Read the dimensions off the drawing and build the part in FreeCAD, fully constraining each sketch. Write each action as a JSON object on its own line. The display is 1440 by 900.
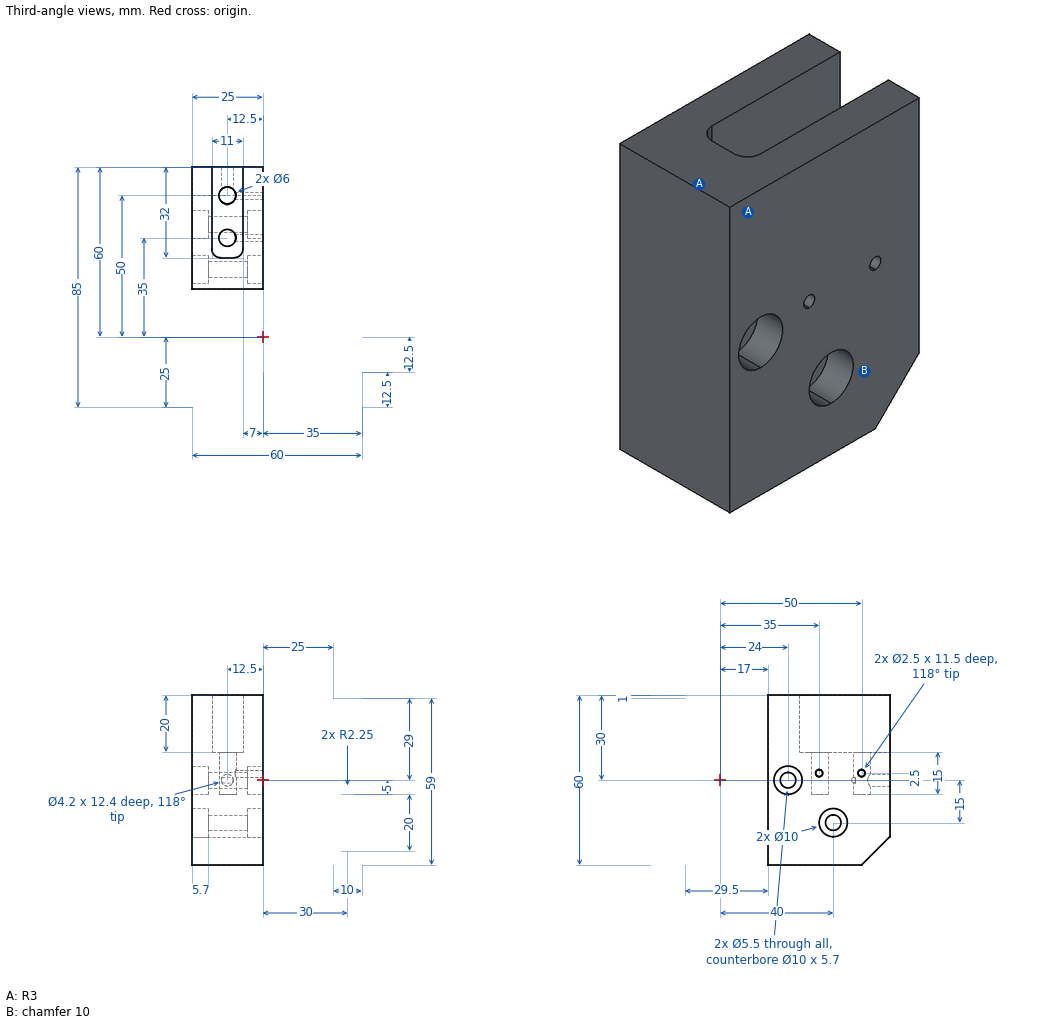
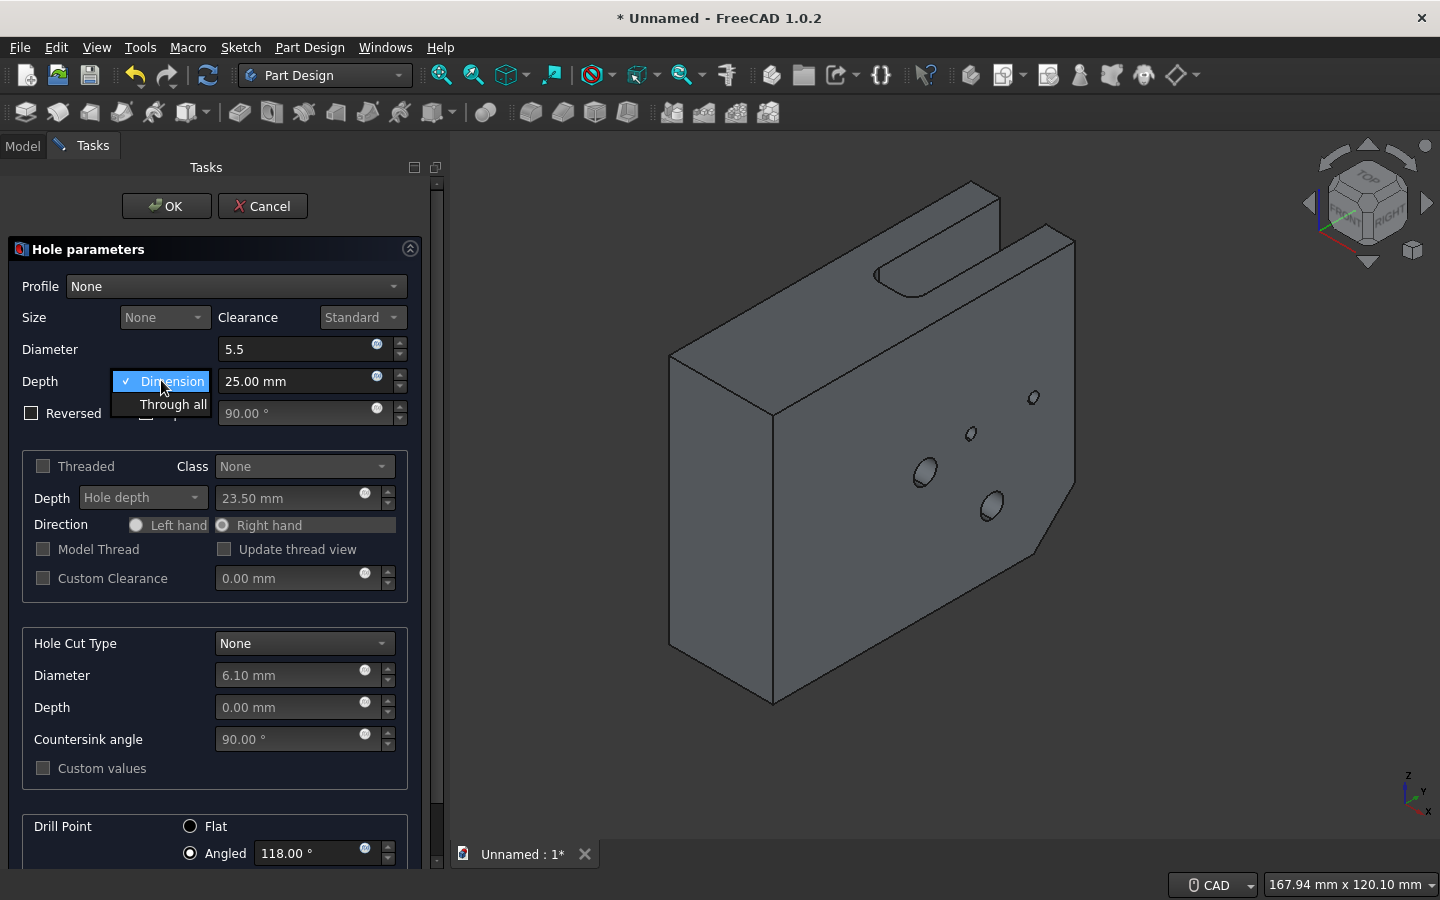
{"action": "left_click", "coordinate": [160, 404]}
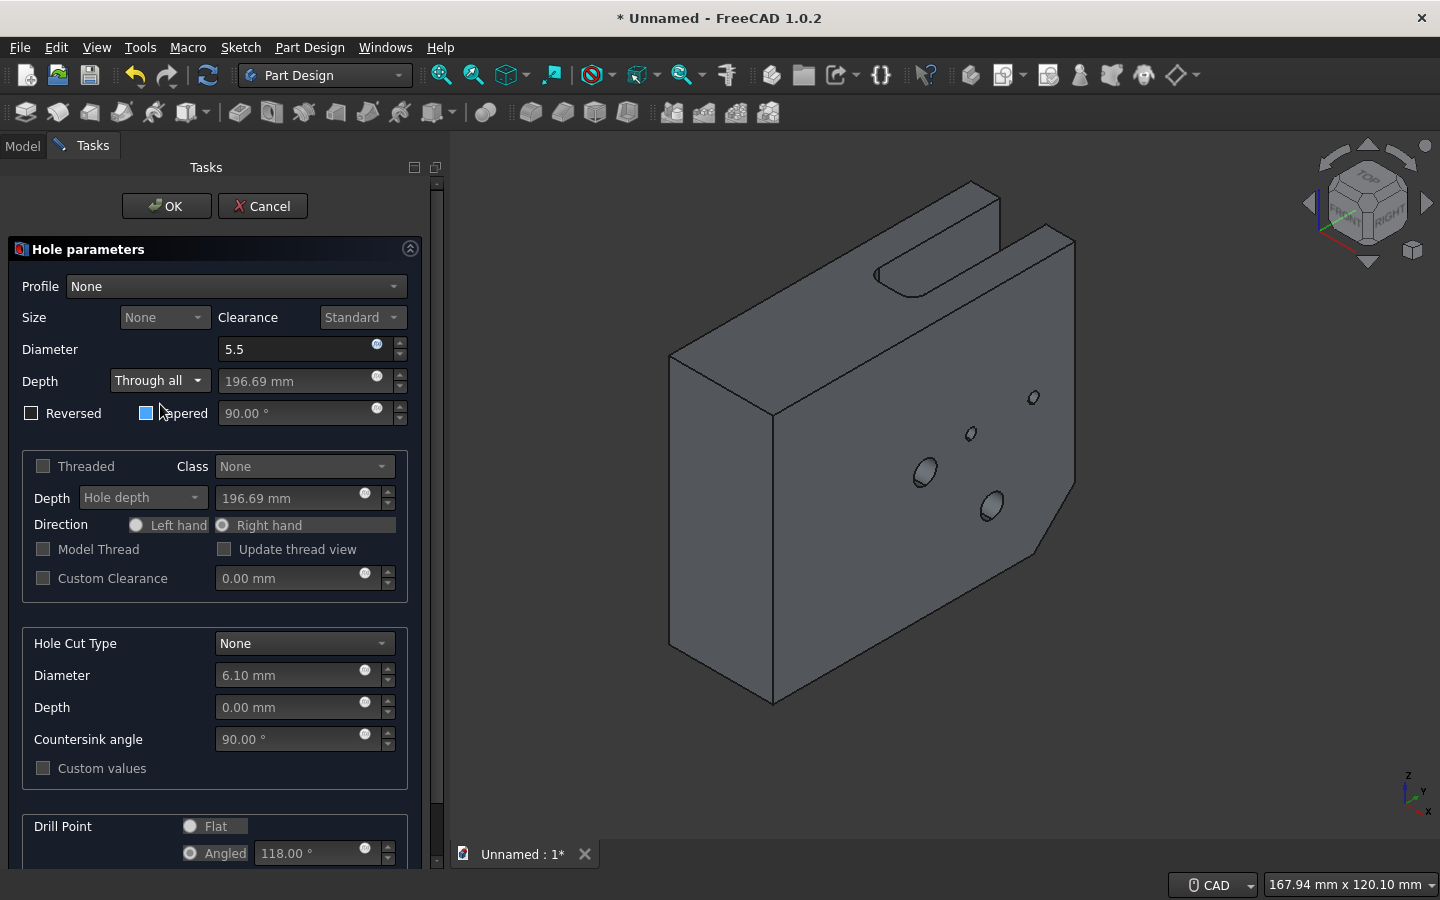
{"action": "left_click", "coordinate": [306, 644]}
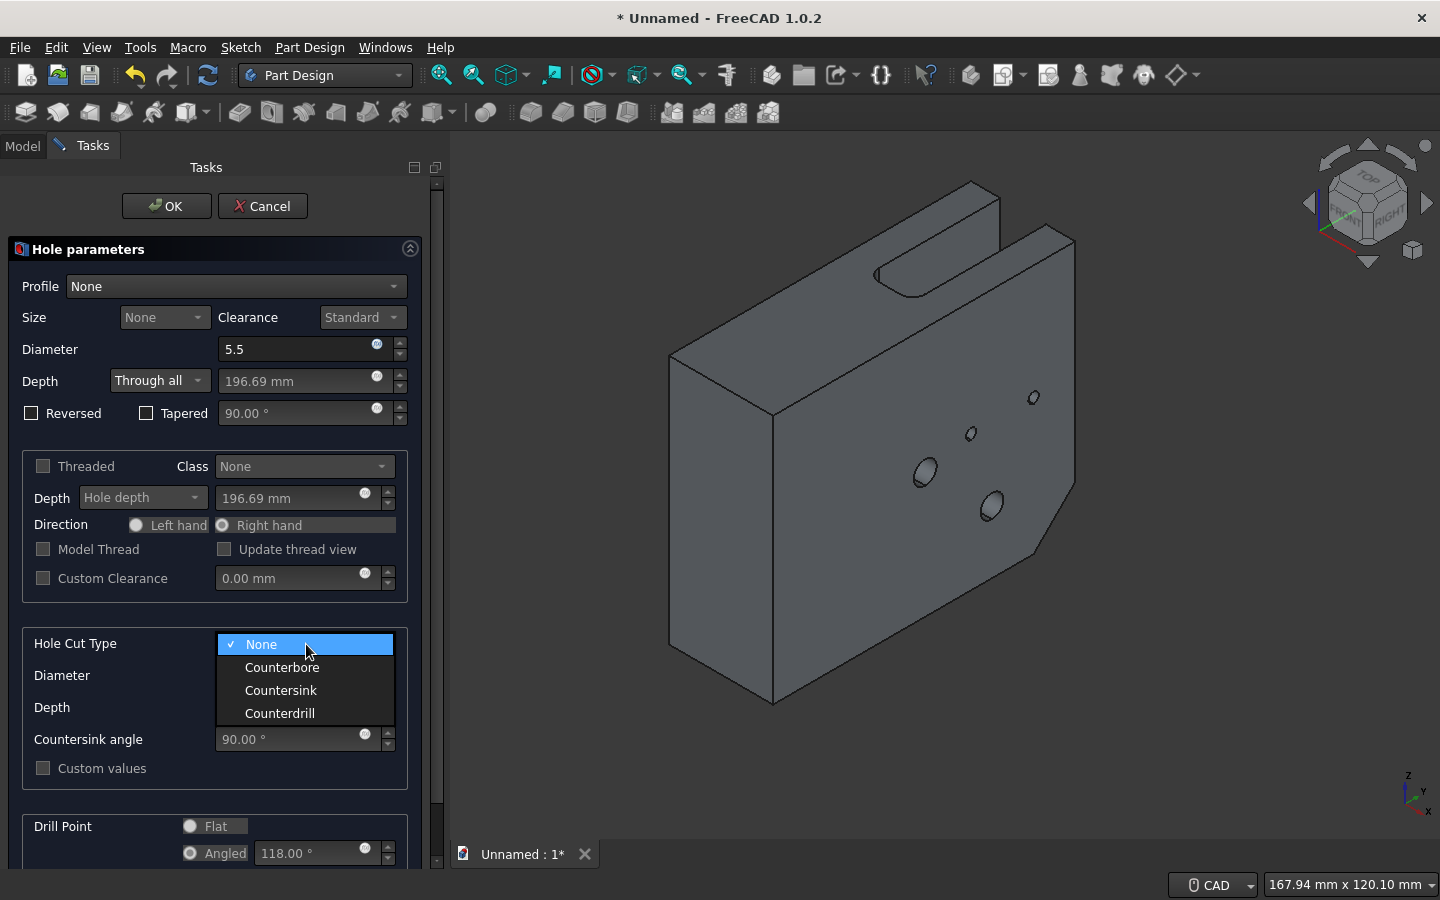
{"action": "left_click", "coordinate": [304, 668]}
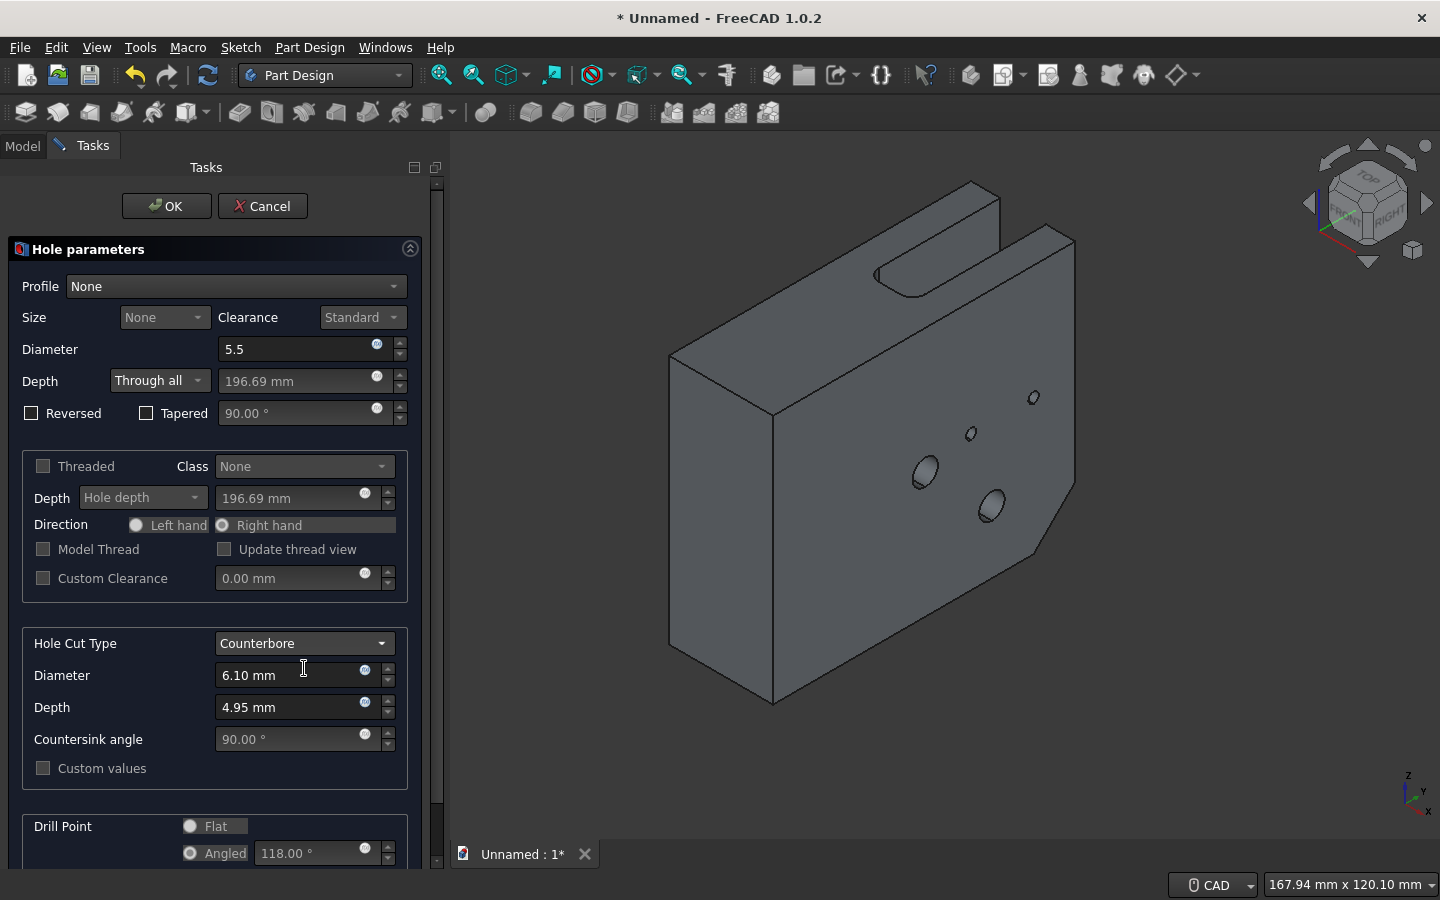
{"action": "triple_click", "coordinate": [298, 675]}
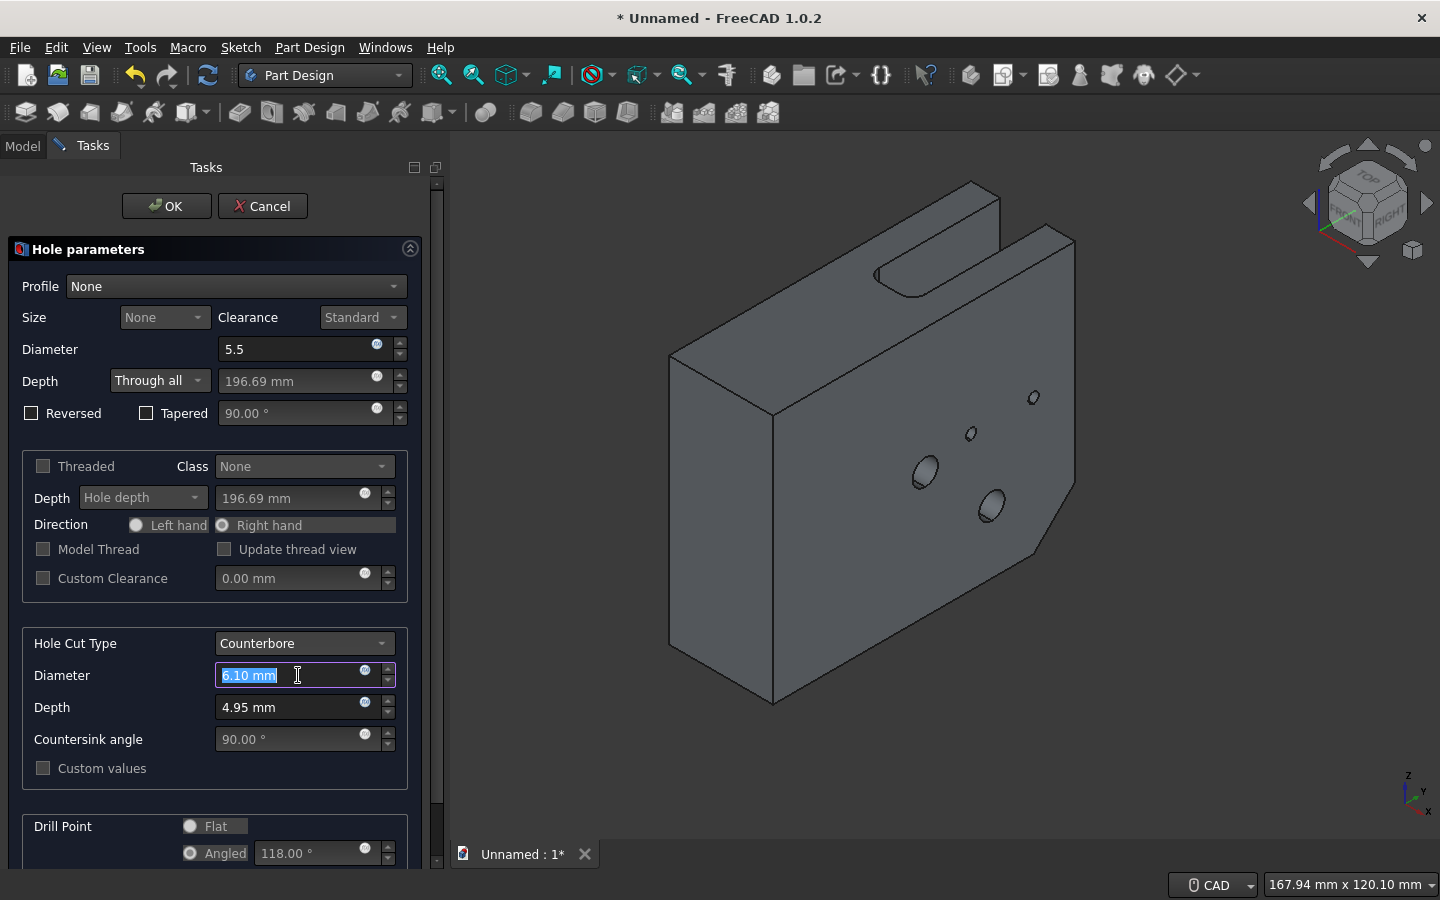
{"action": "type", "text": "10"}
{"action": "key", "text": "Tab"}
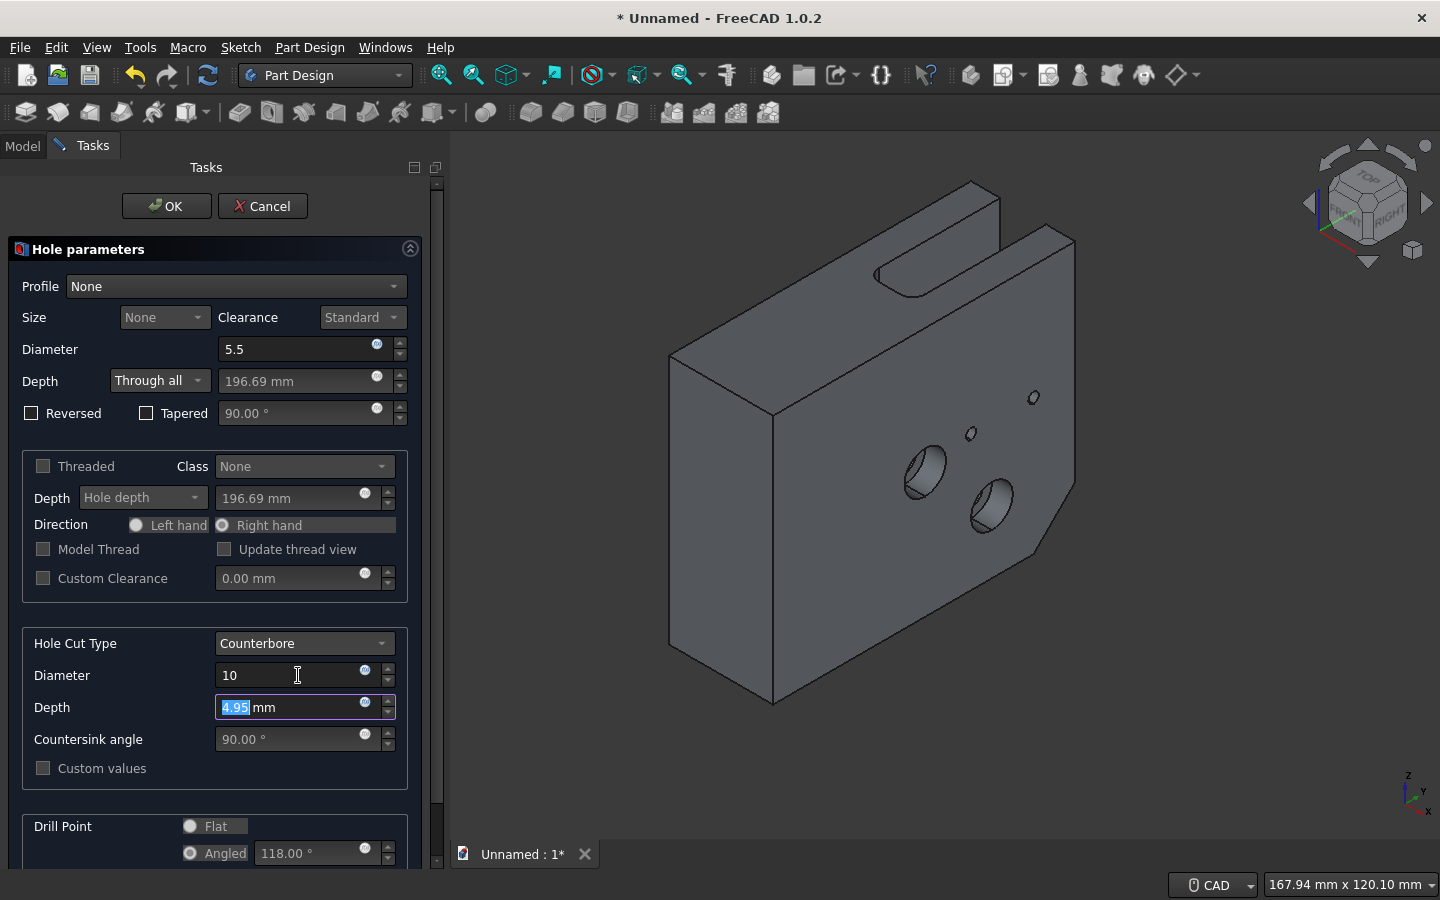
{"action": "type", "text": "5.7"}
{"action": "key", "text": "Tab"}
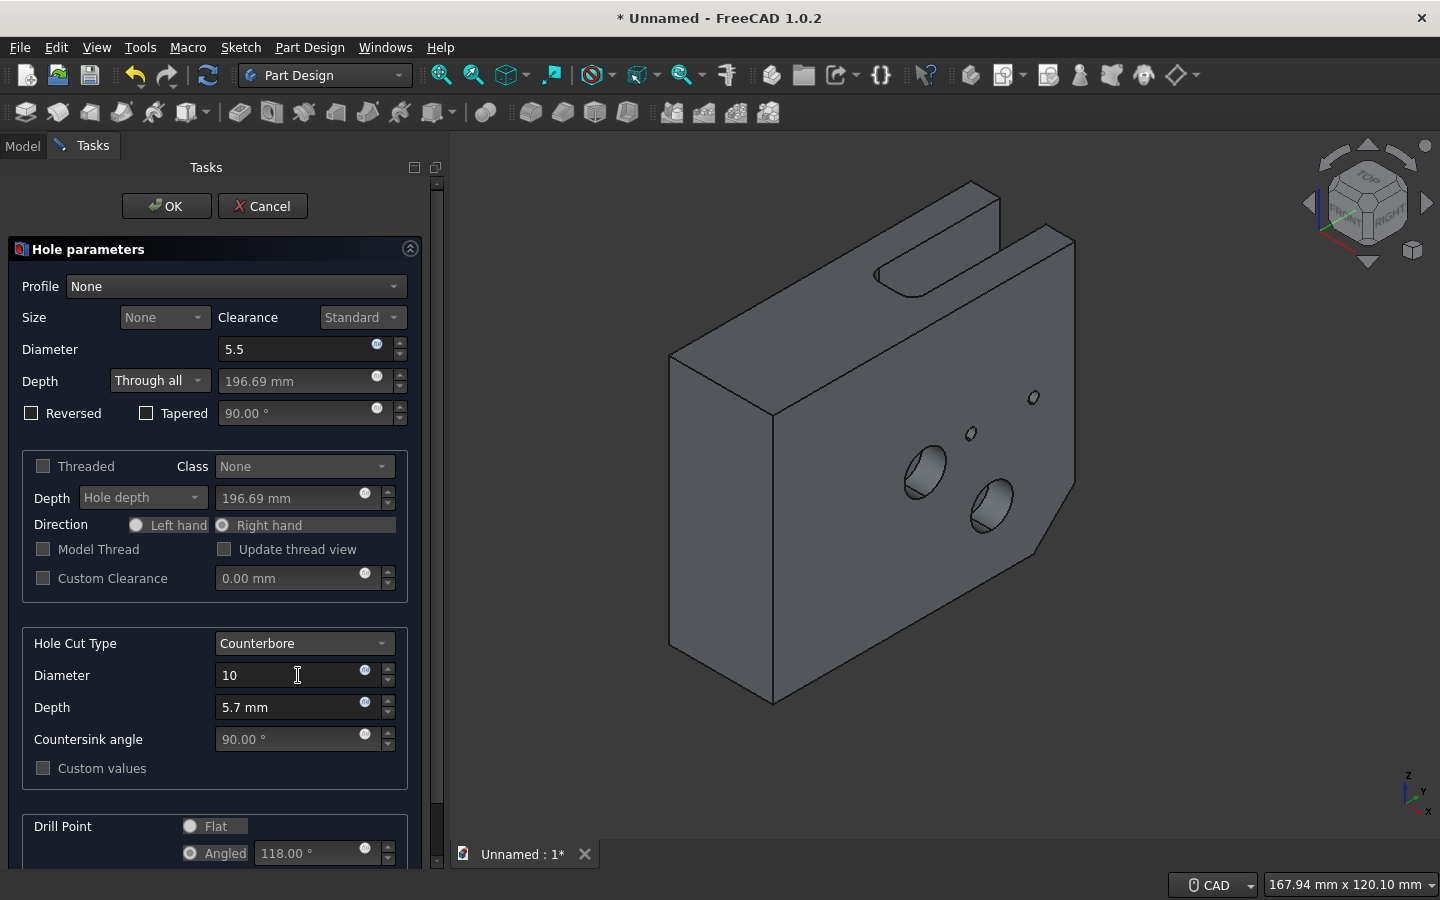
{"action": "left_click", "coordinate": [167, 206]}